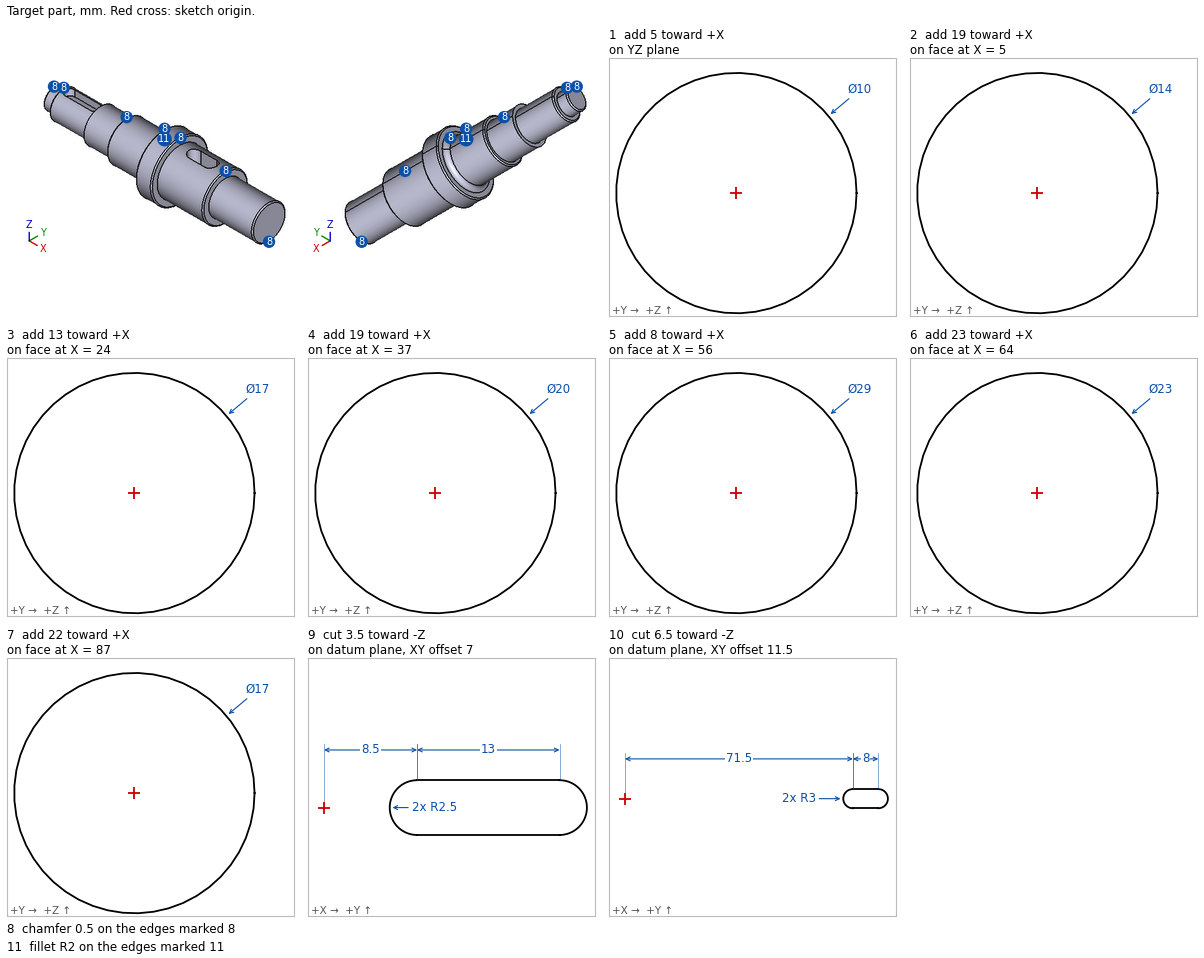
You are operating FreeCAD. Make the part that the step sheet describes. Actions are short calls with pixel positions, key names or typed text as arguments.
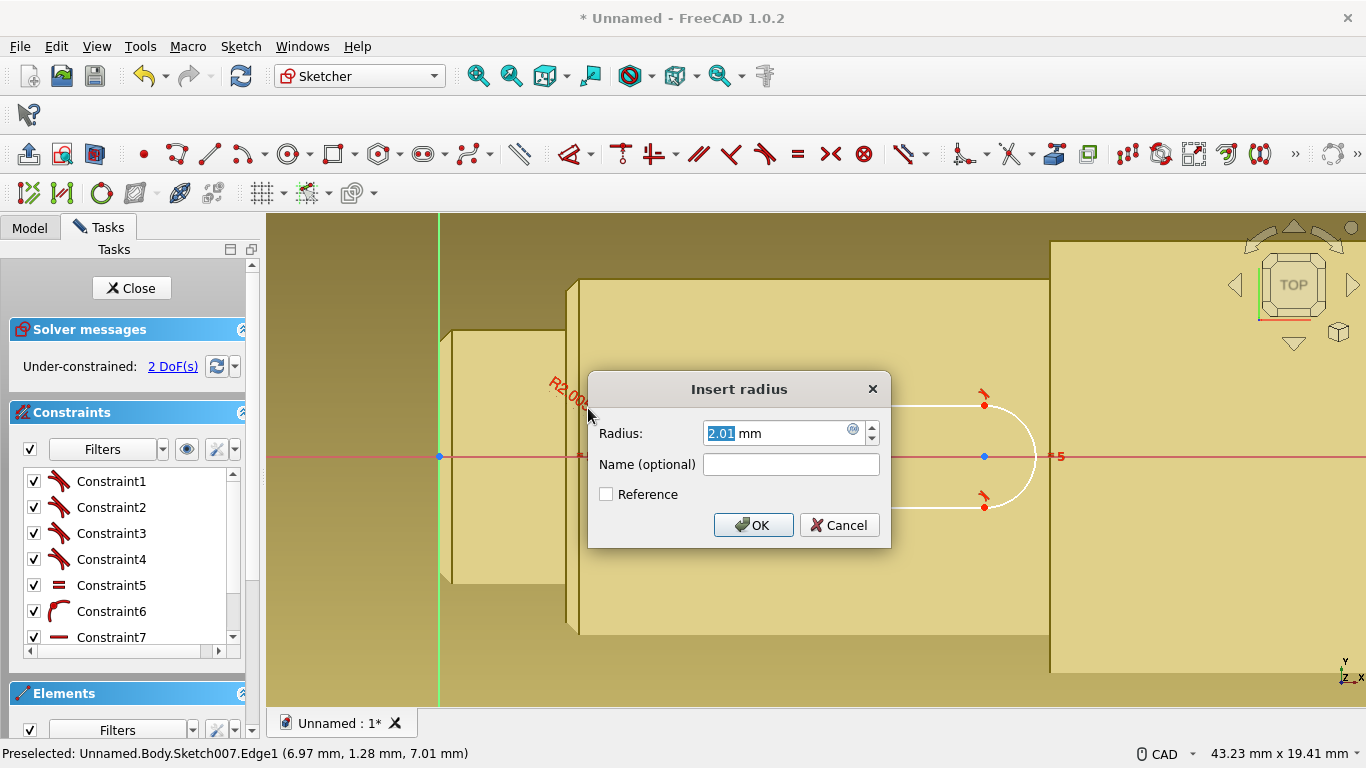
text(2.5)
key(Return)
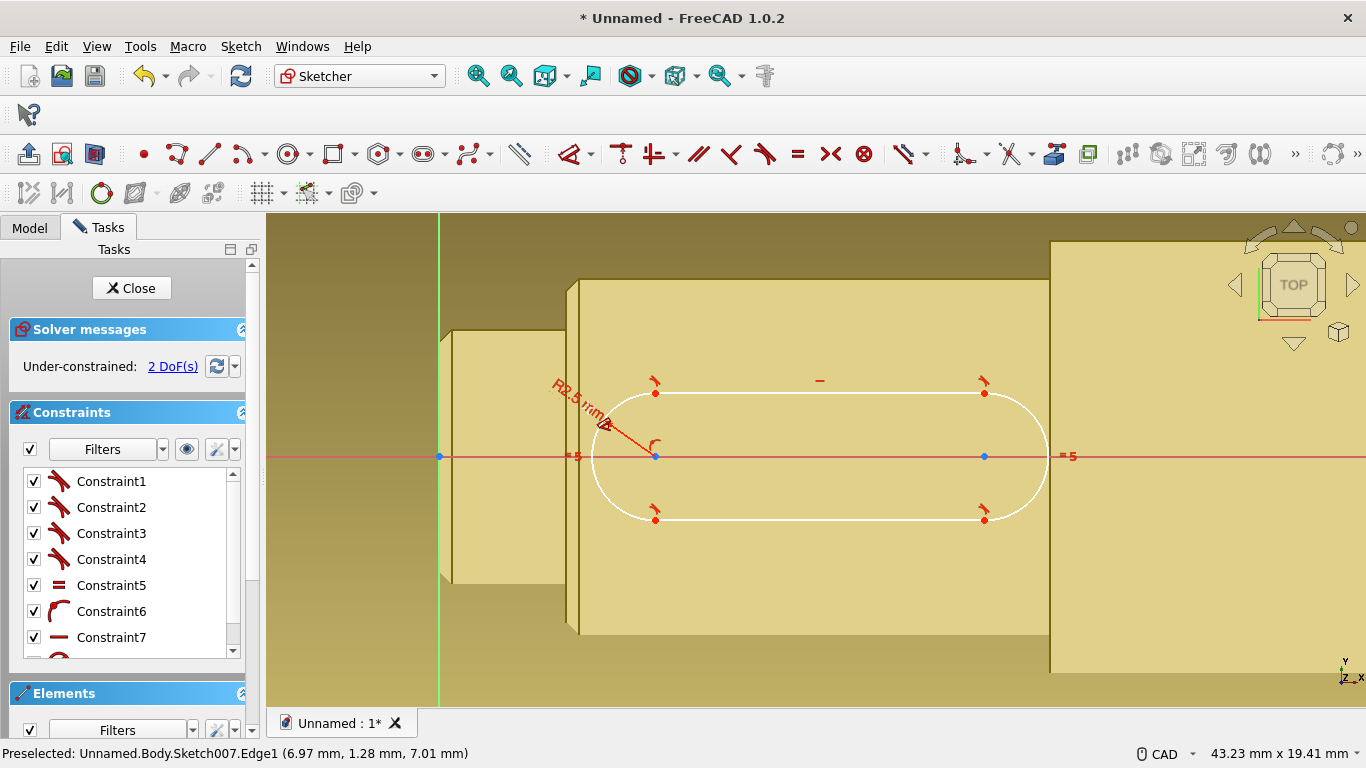
click(754, 393)
click(820, 359)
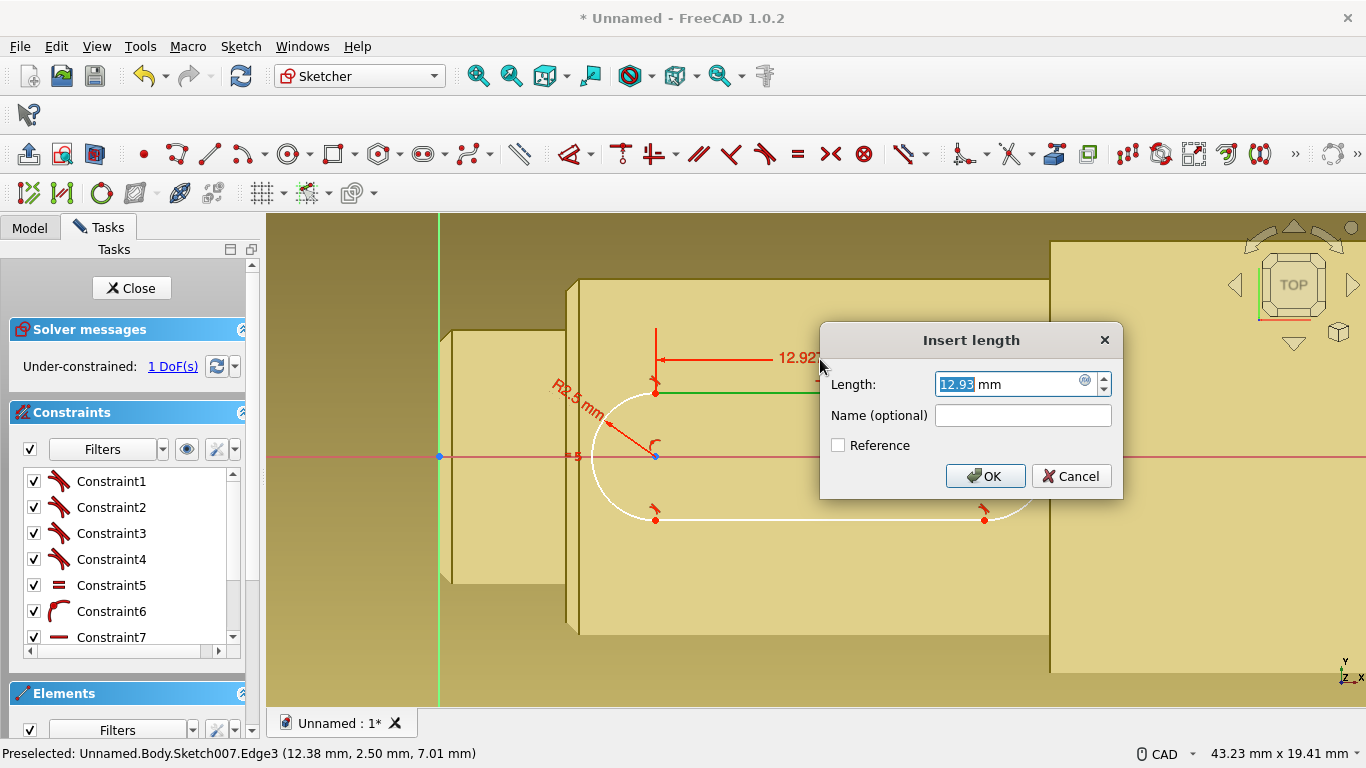
text(13)
key(Return)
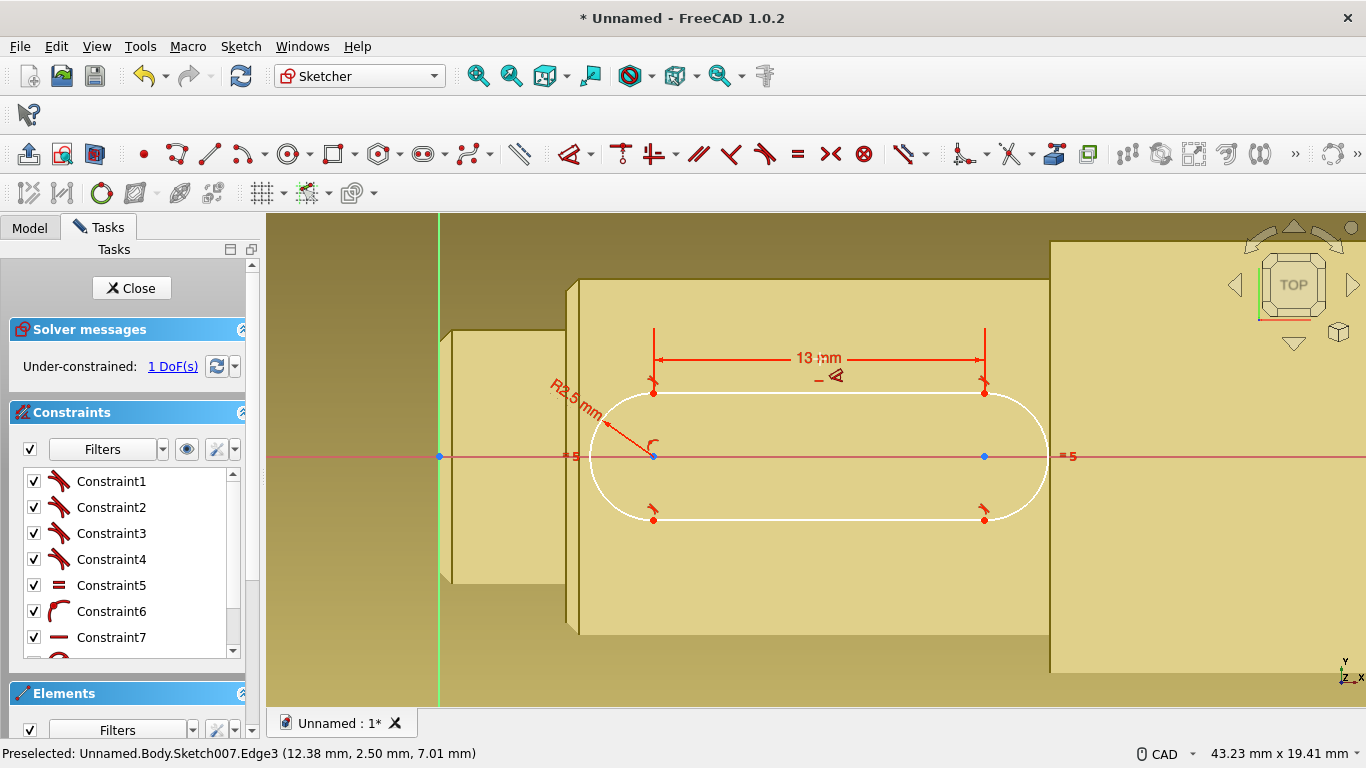
click(654, 393)
click(546, 359)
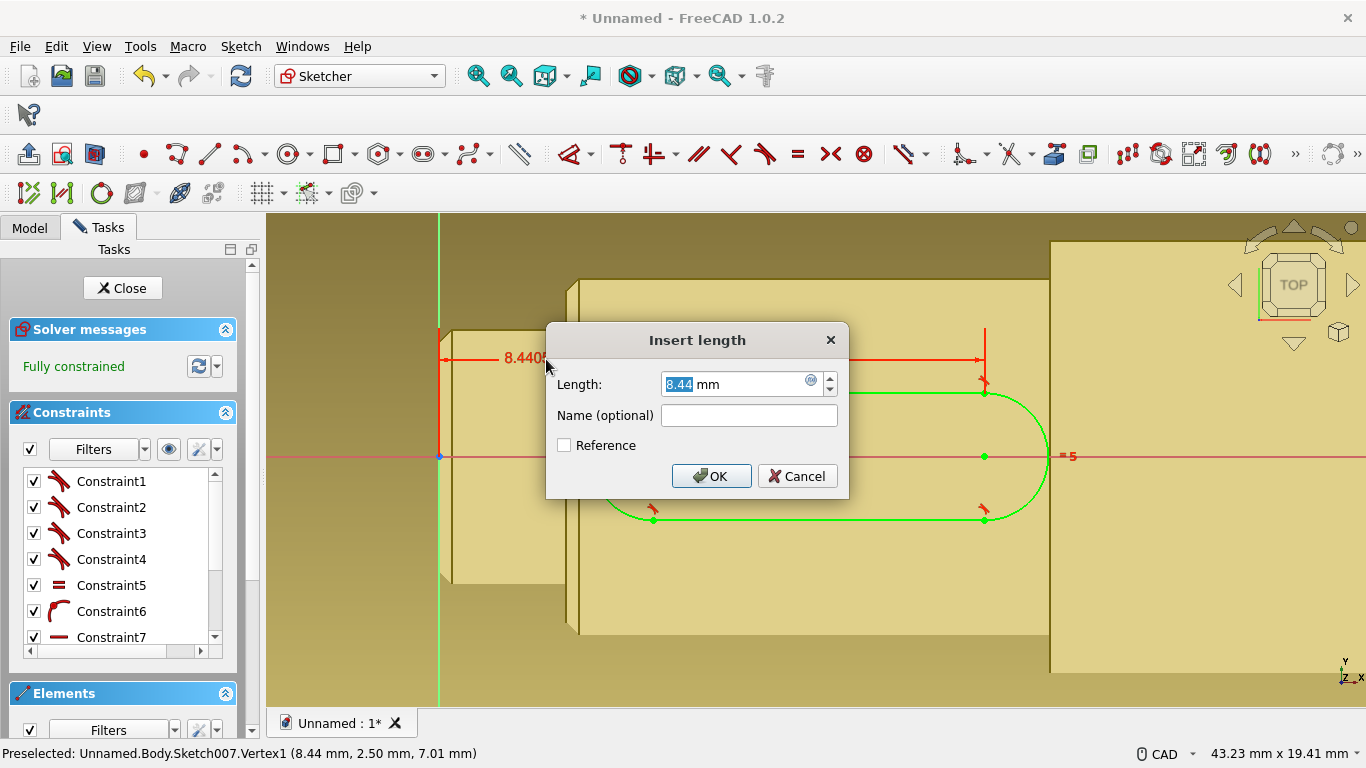
text(8.5)
key(Return)
key(Escape)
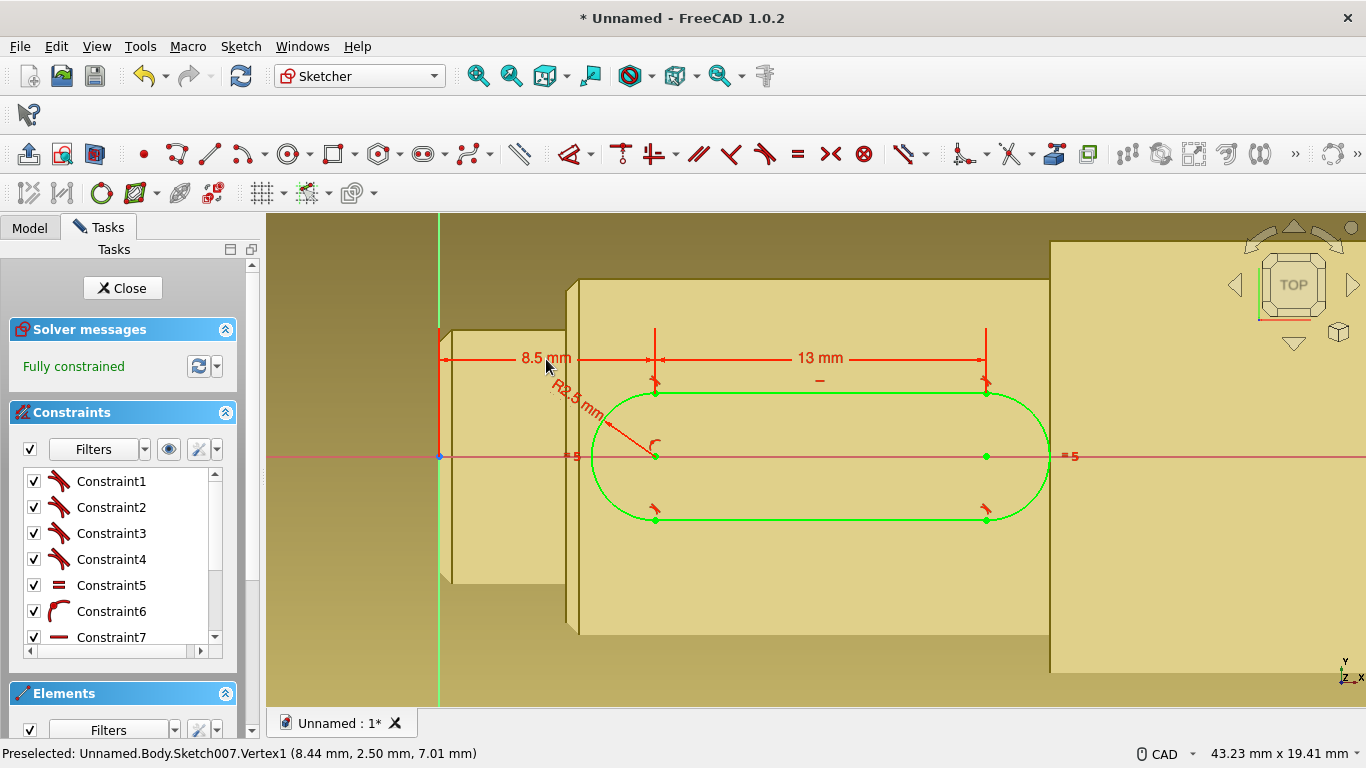
click(123, 288)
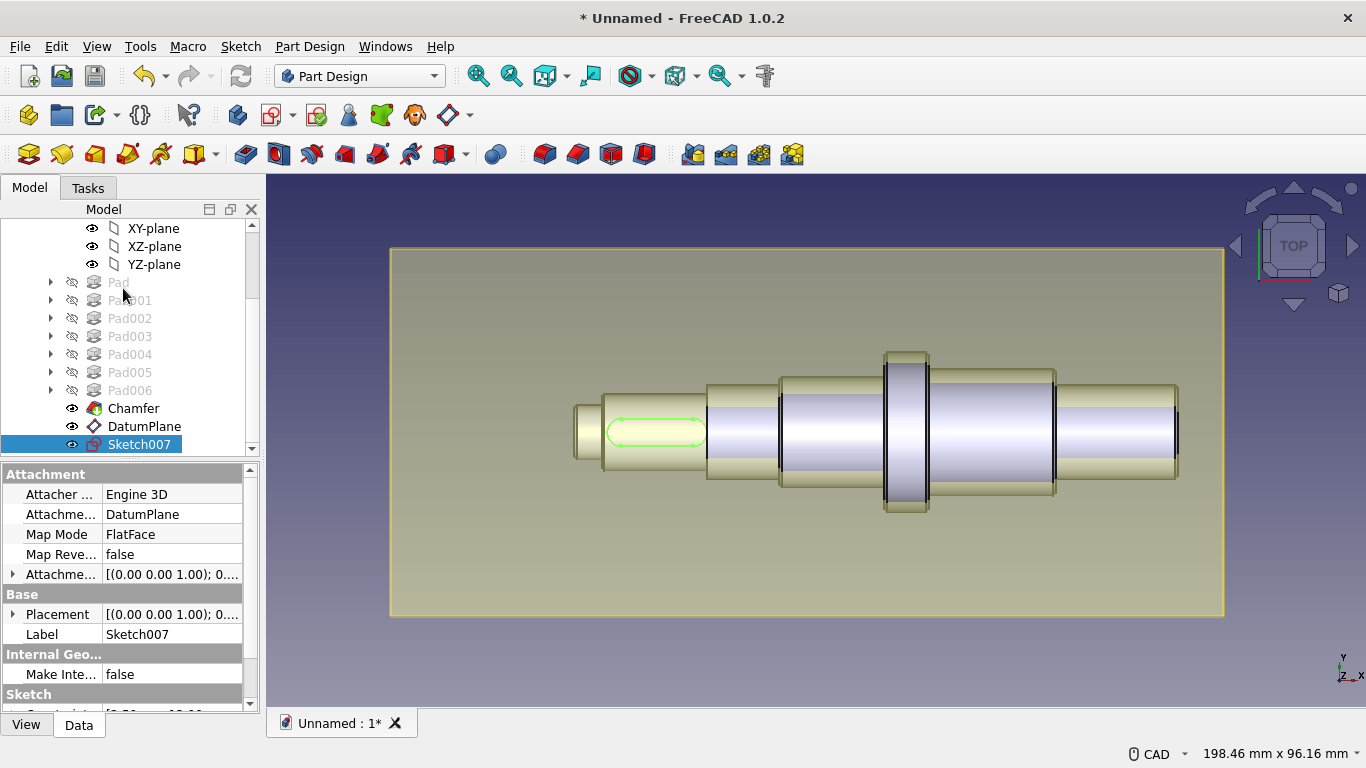
click(246, 154)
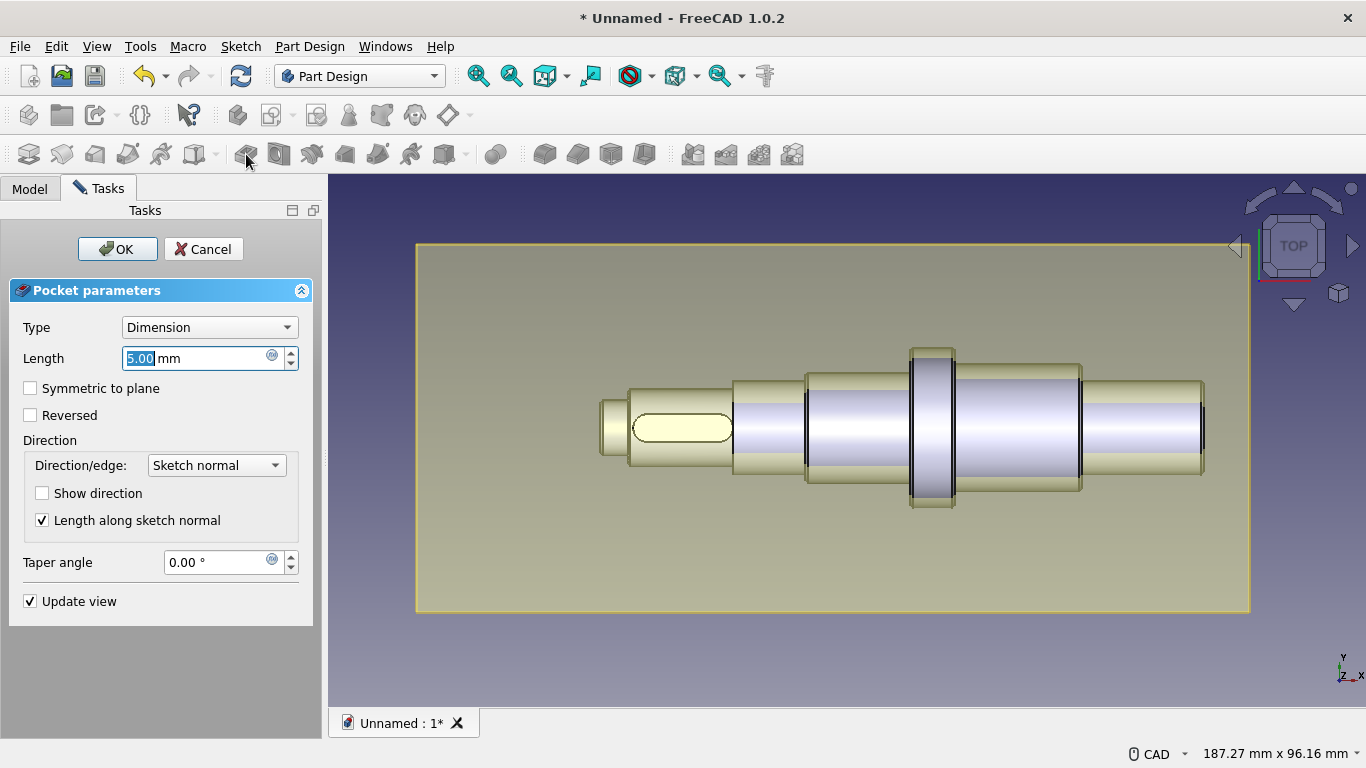
text(3.5)
key(Tab)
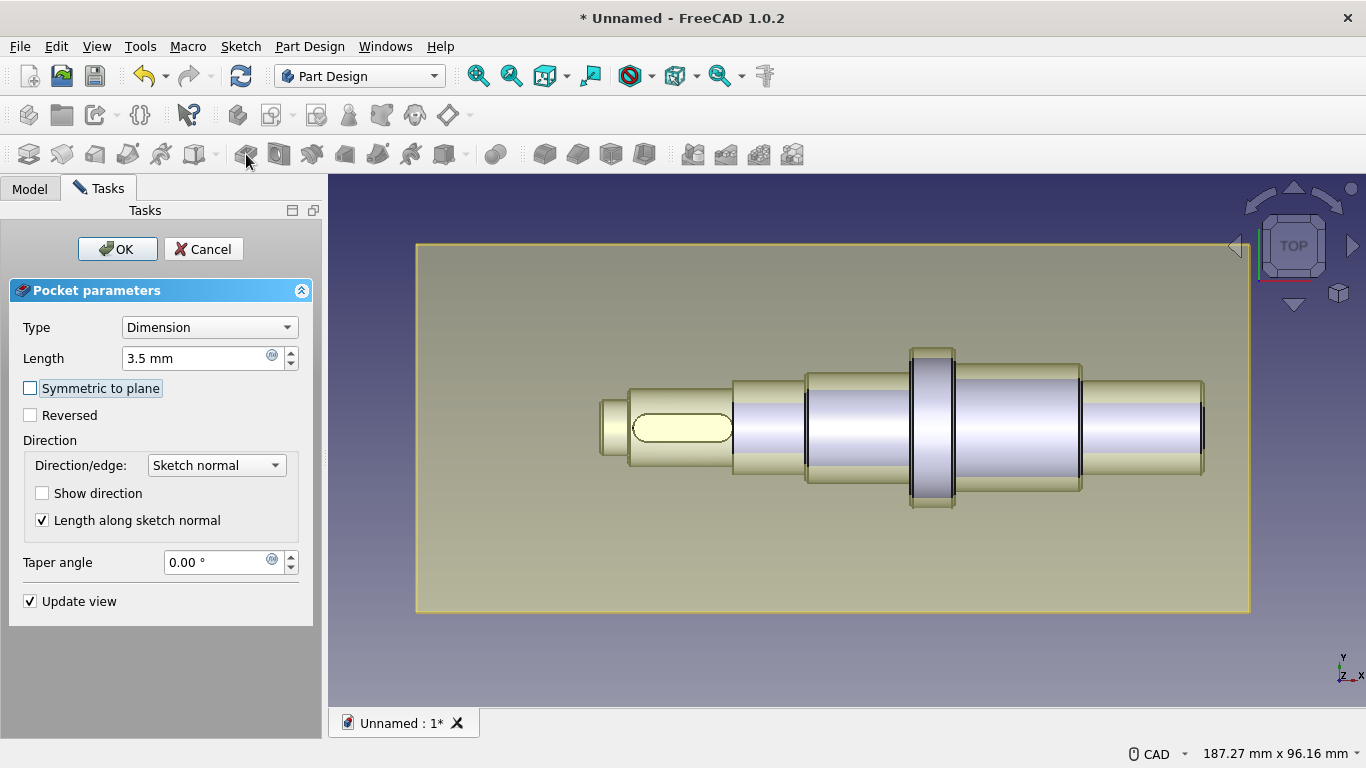
click(118, 249)